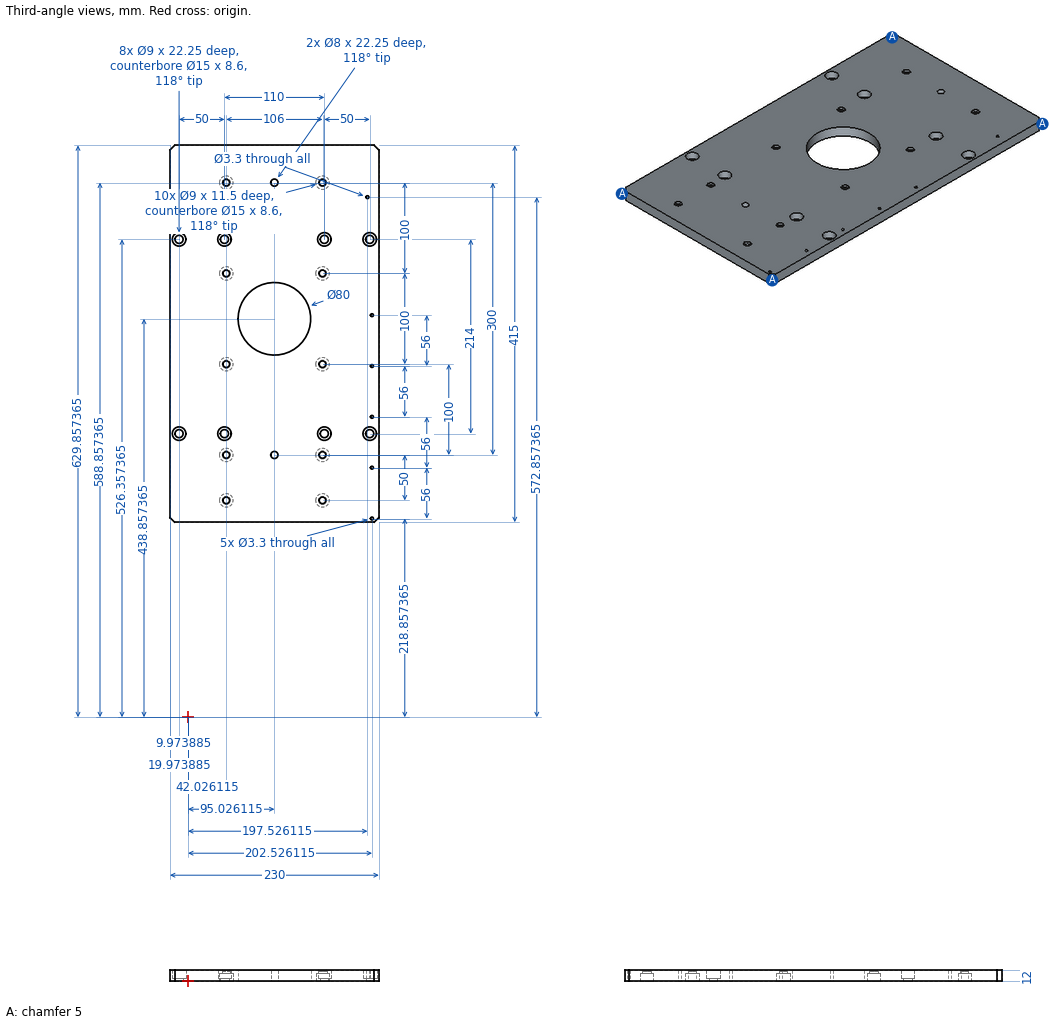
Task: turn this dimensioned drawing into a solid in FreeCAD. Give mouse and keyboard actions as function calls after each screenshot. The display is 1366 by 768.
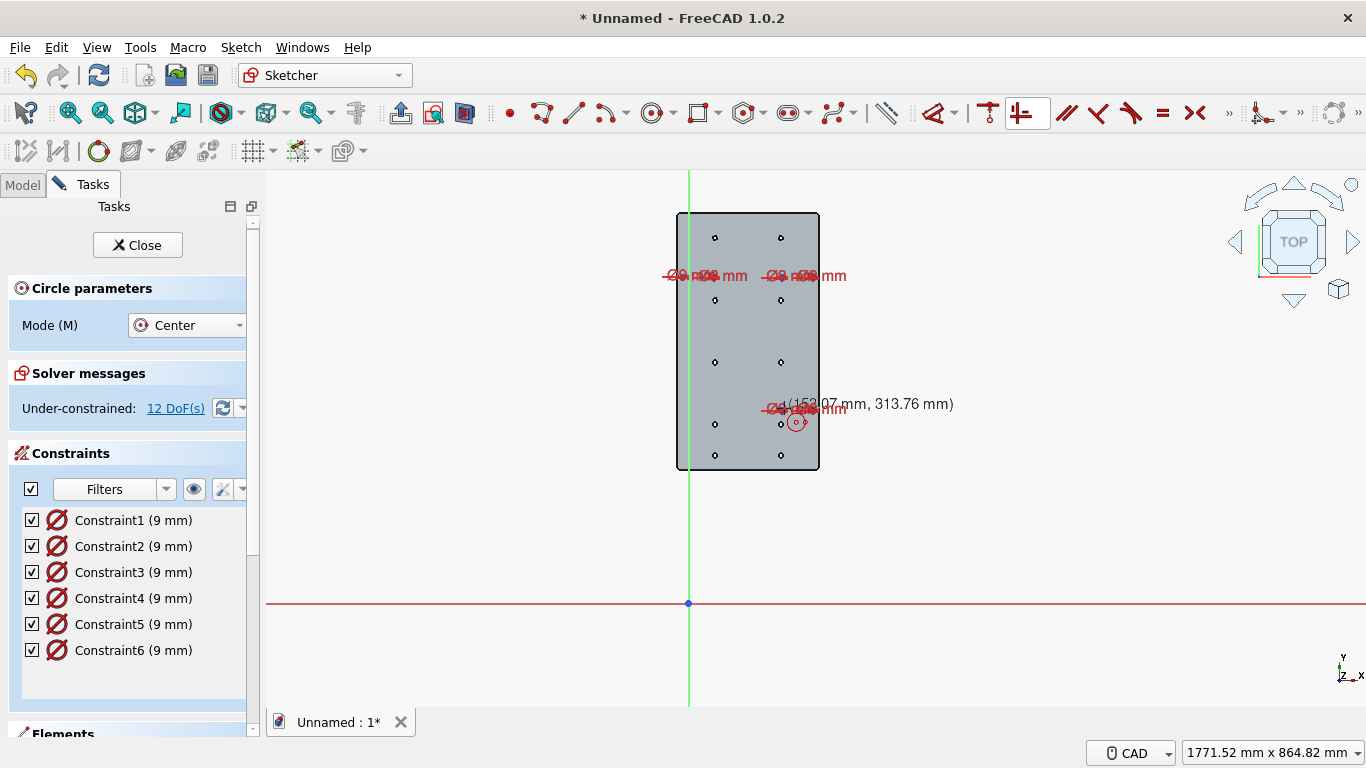
scroll(714, 410, up, 11)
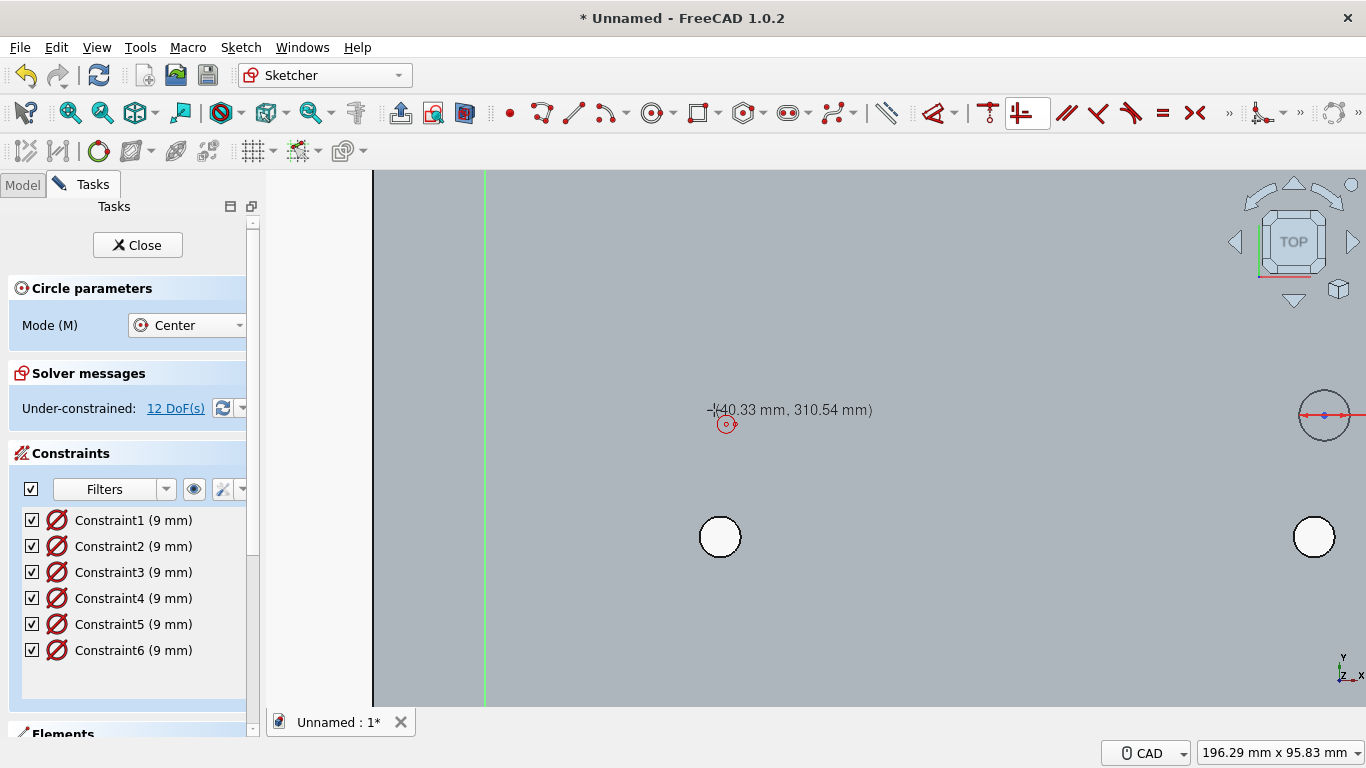
scroll(714, 410, down, 11)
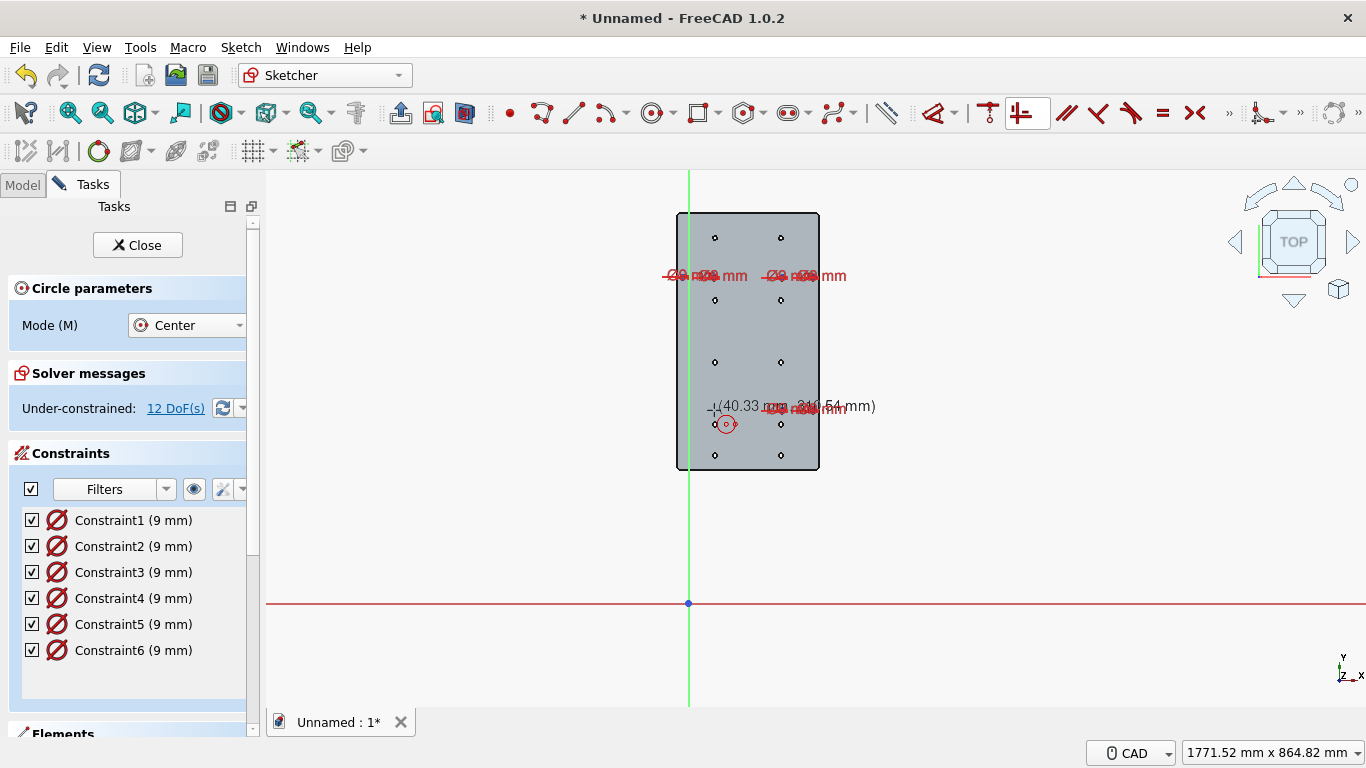
click(714, 410)
move(716, 408)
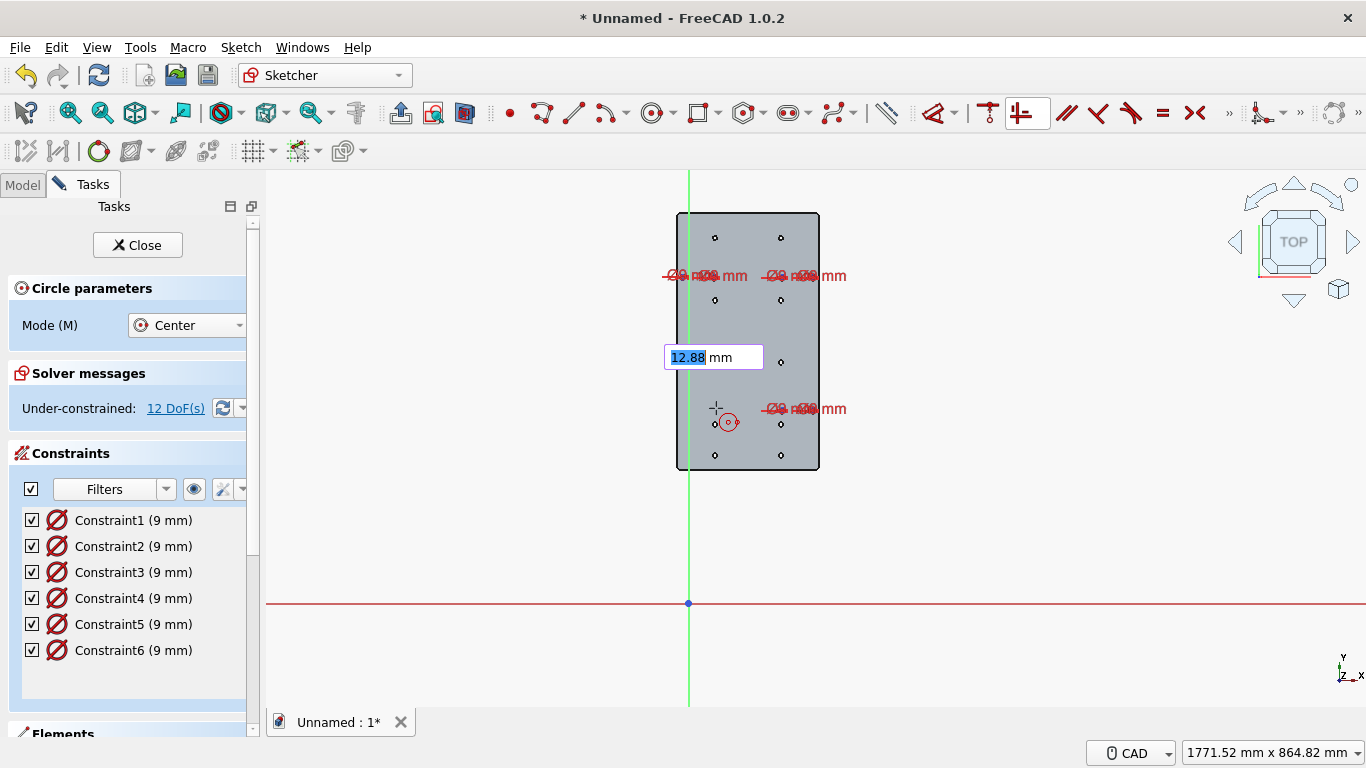
text(9)
key(Return)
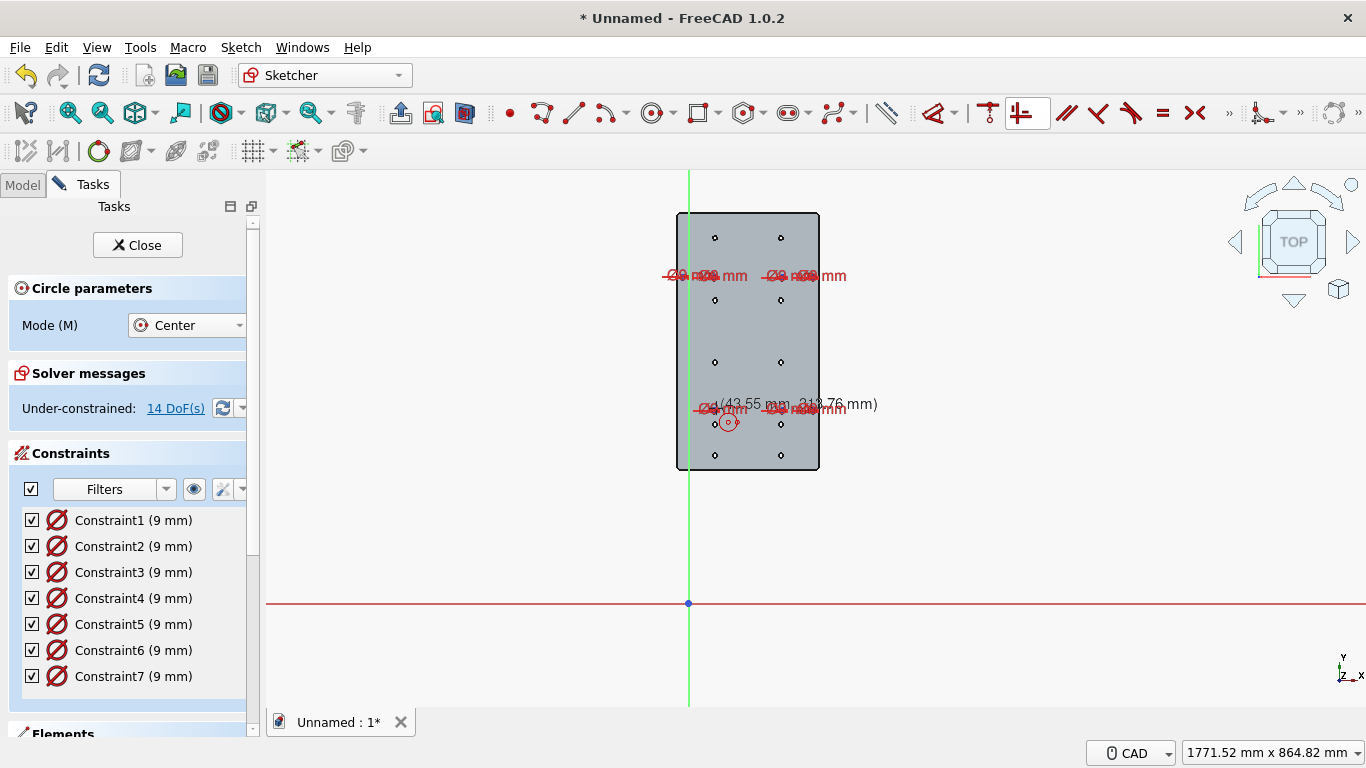
scroll(683, 410, up, 11)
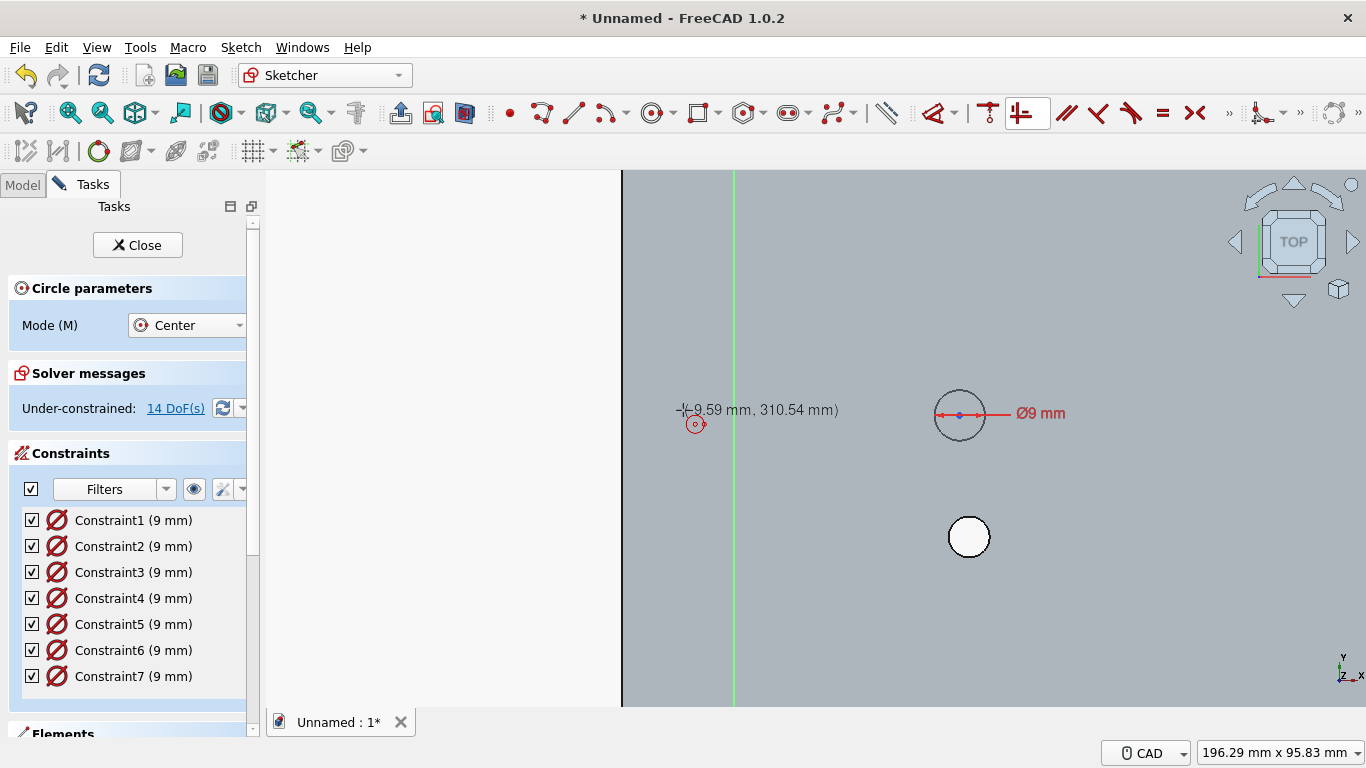
scroll(683, 410, down, 11)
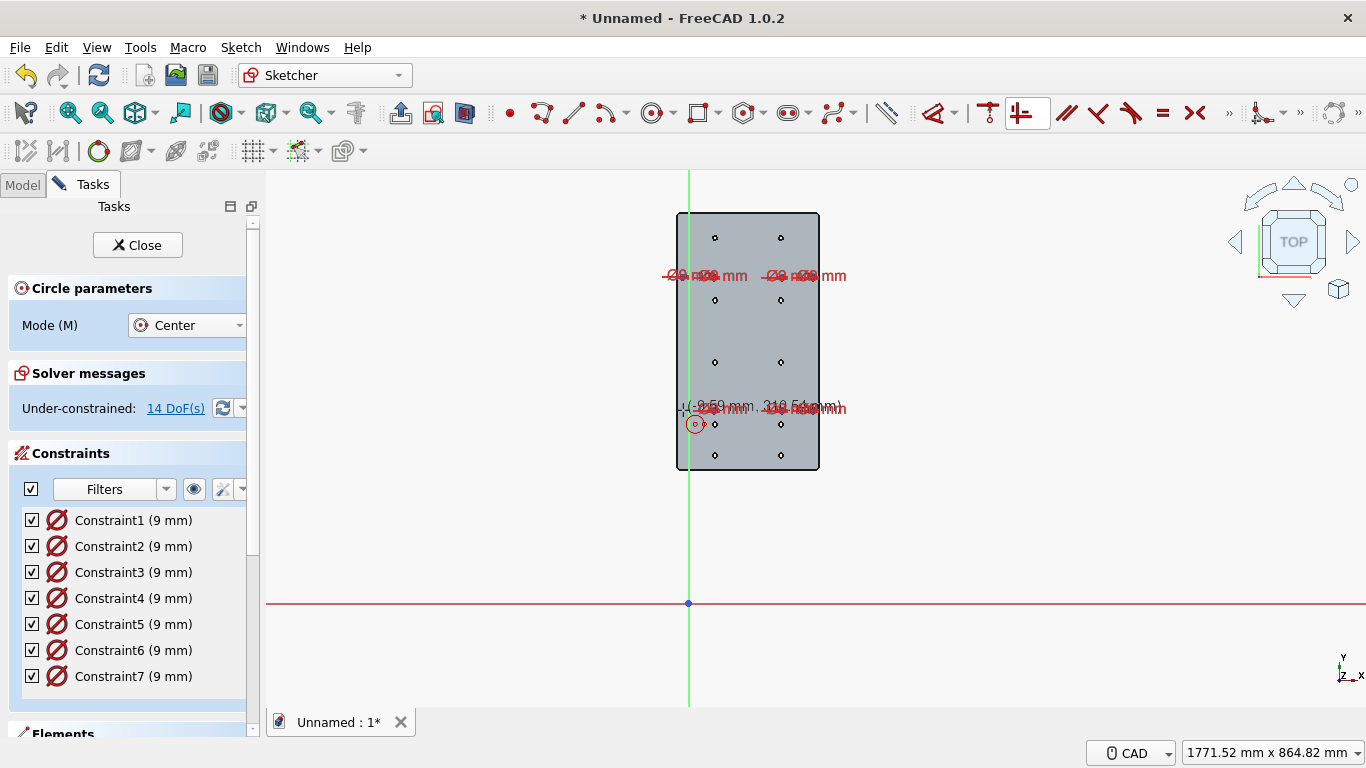
scroll(683, 410, up, 5)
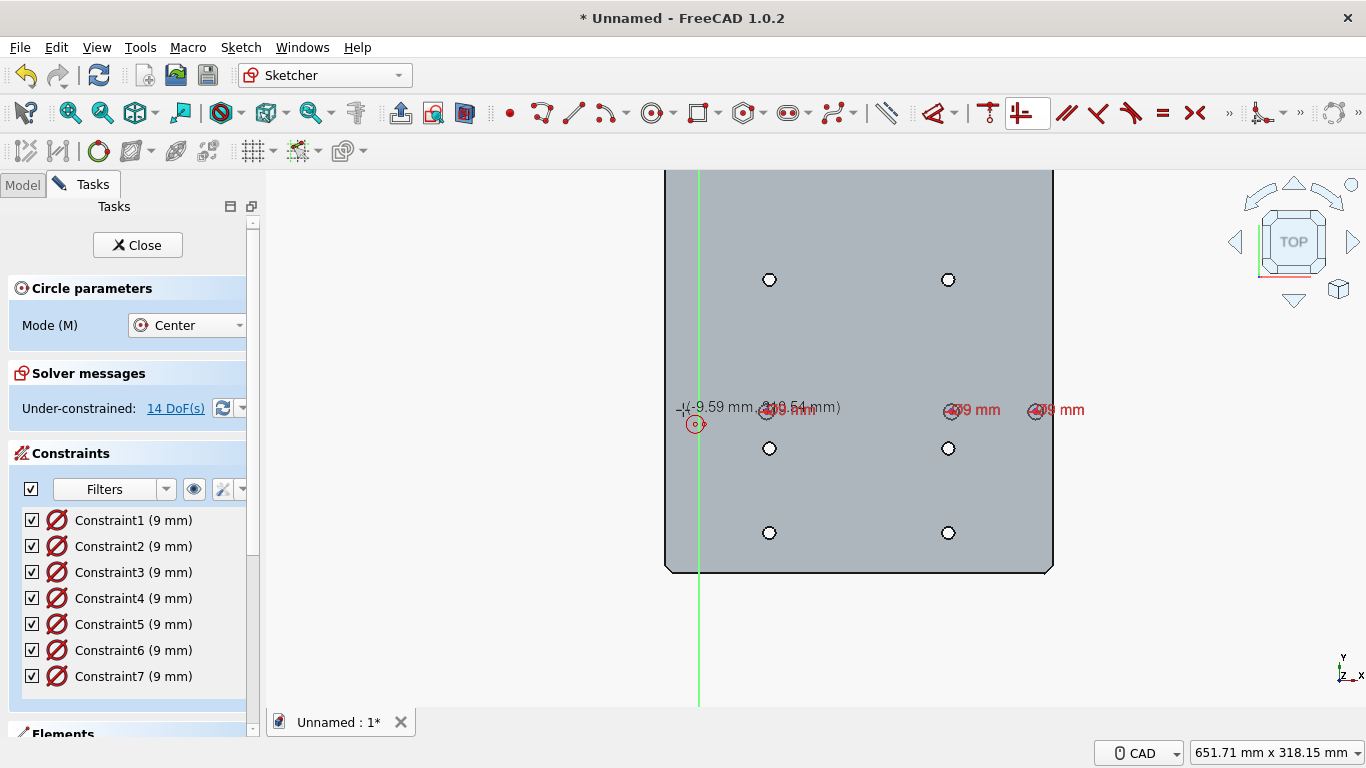
click(682, 409)
move(676, 404)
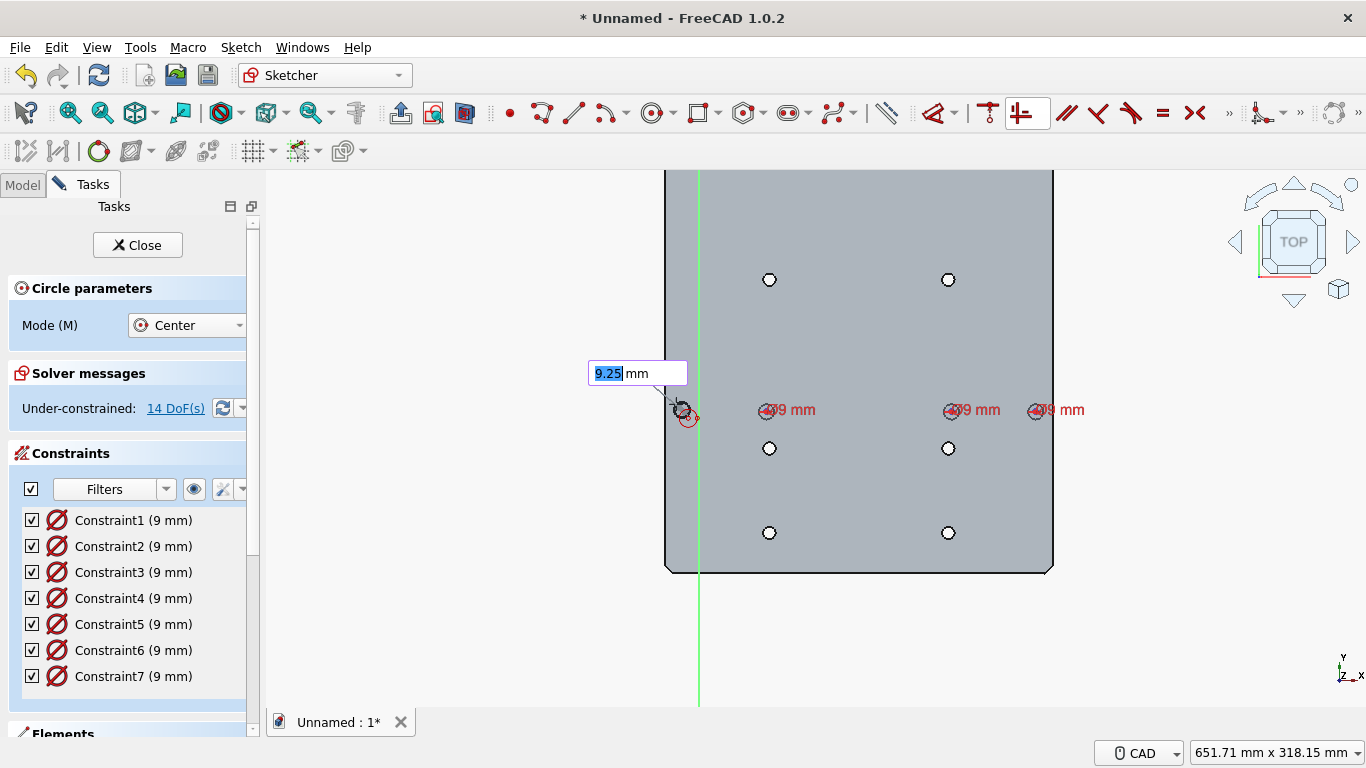
text(9)
key(Return)
key(Escape)